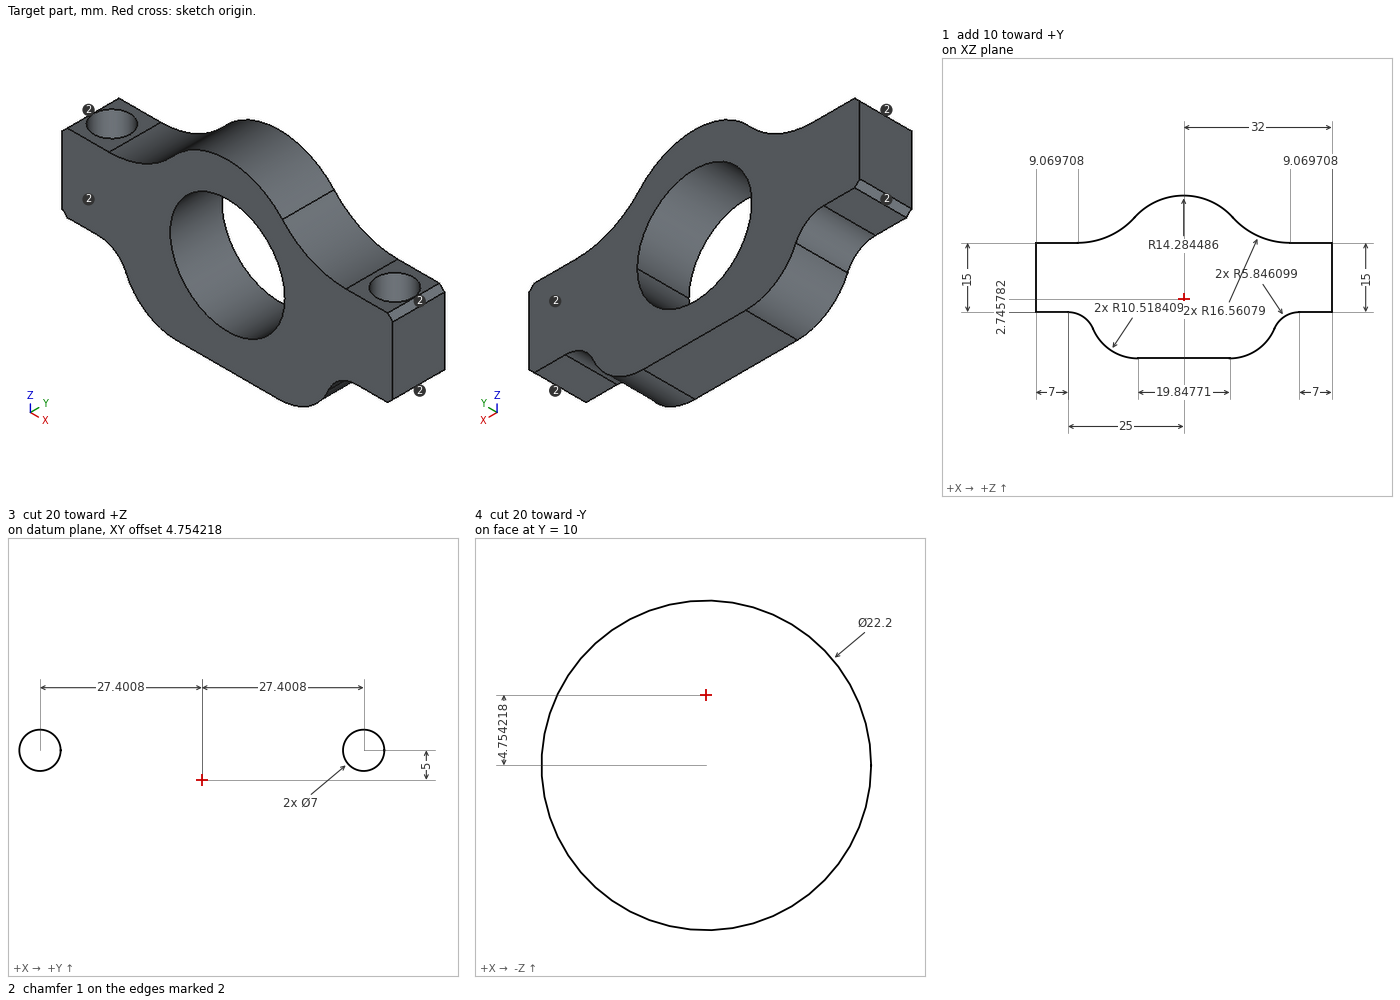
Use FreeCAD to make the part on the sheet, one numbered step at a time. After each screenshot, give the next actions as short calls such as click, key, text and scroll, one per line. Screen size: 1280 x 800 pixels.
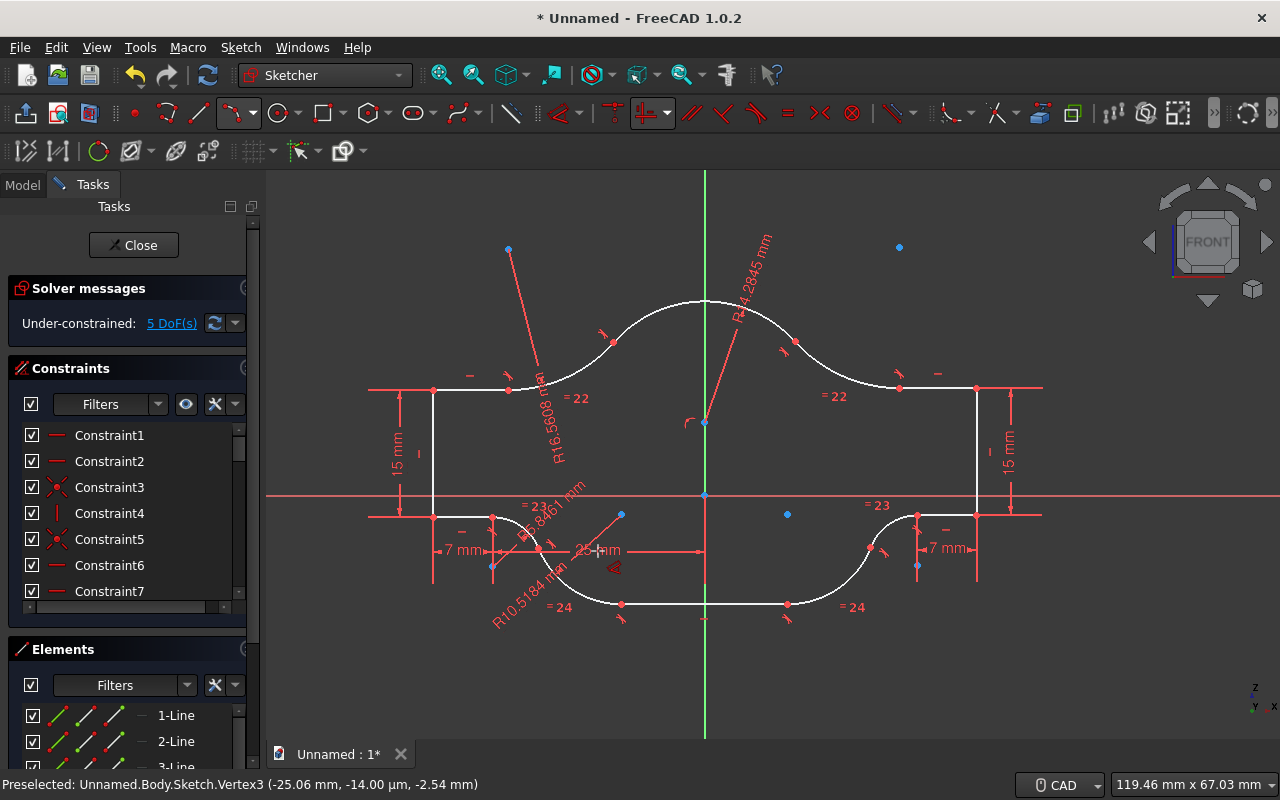
click(977, 388)
click(841, 354)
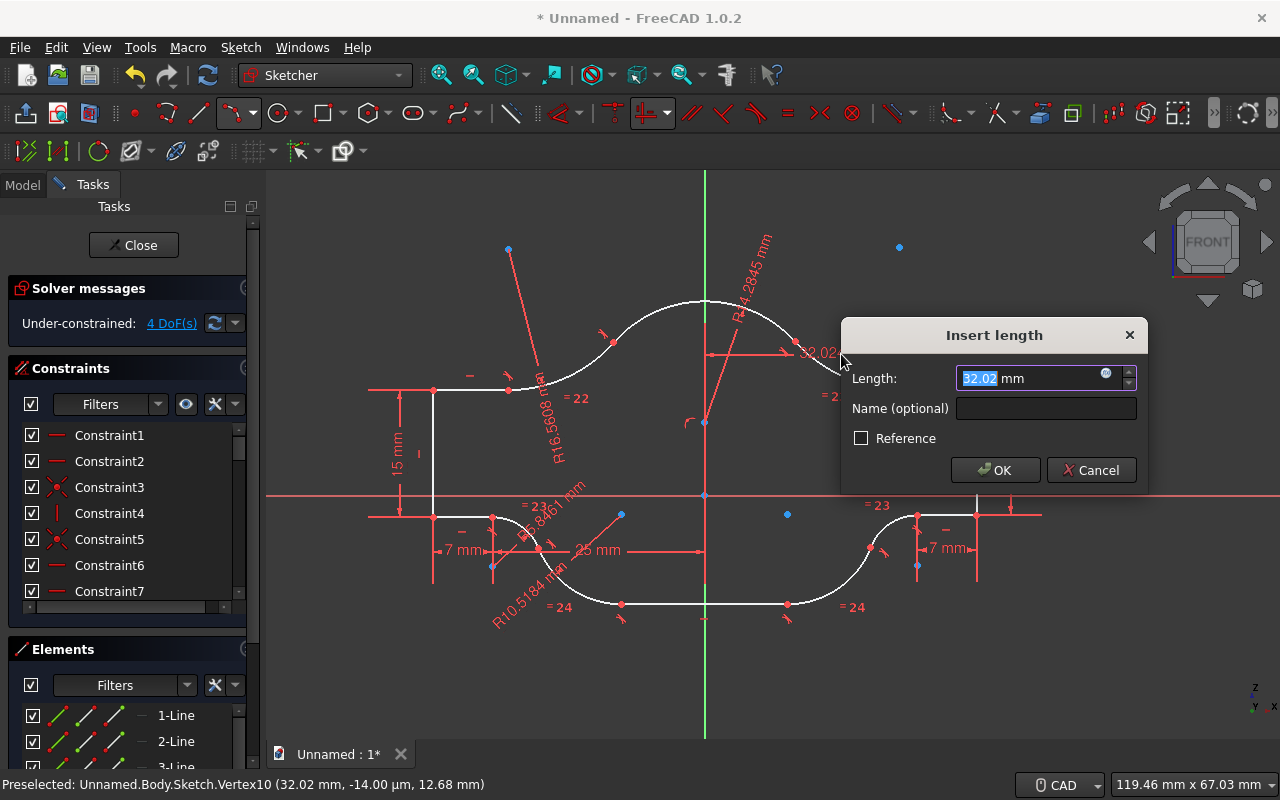
text(32)
key(Return)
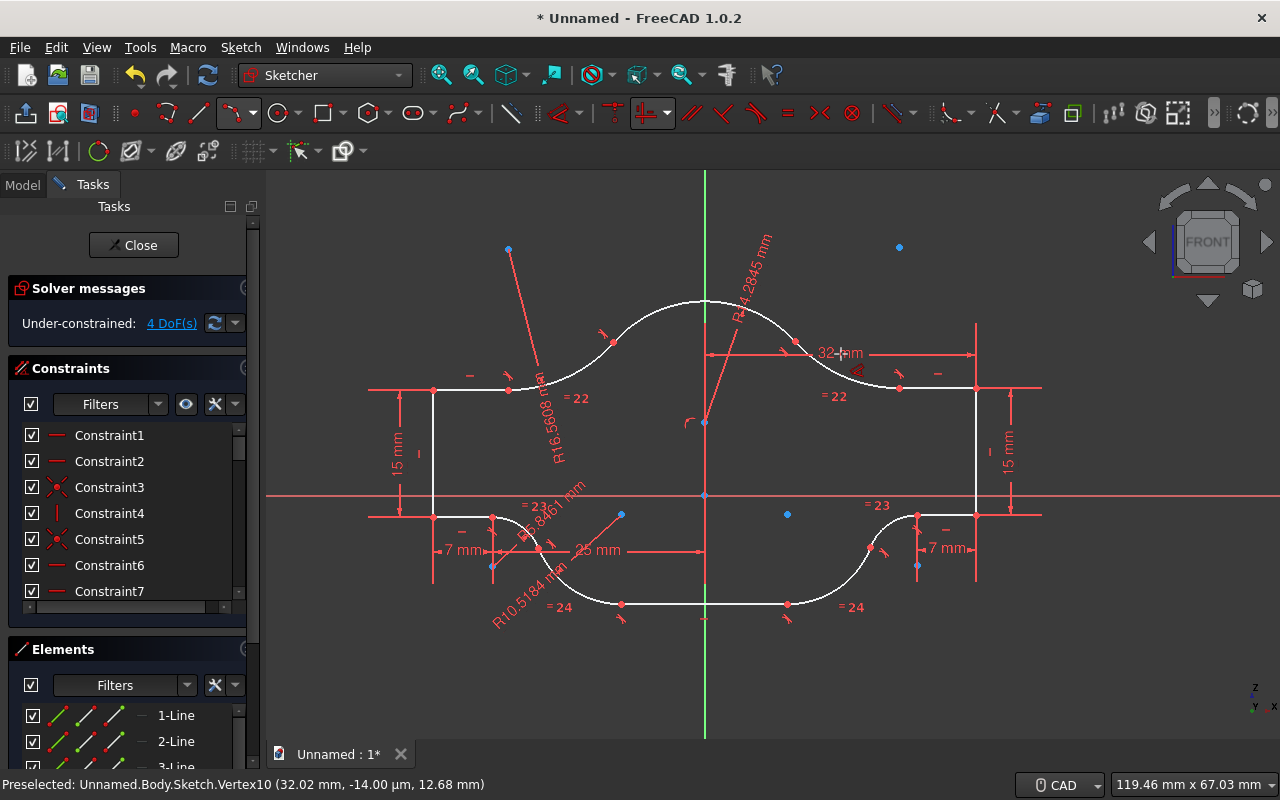
click(738, 604)
click(666, 638)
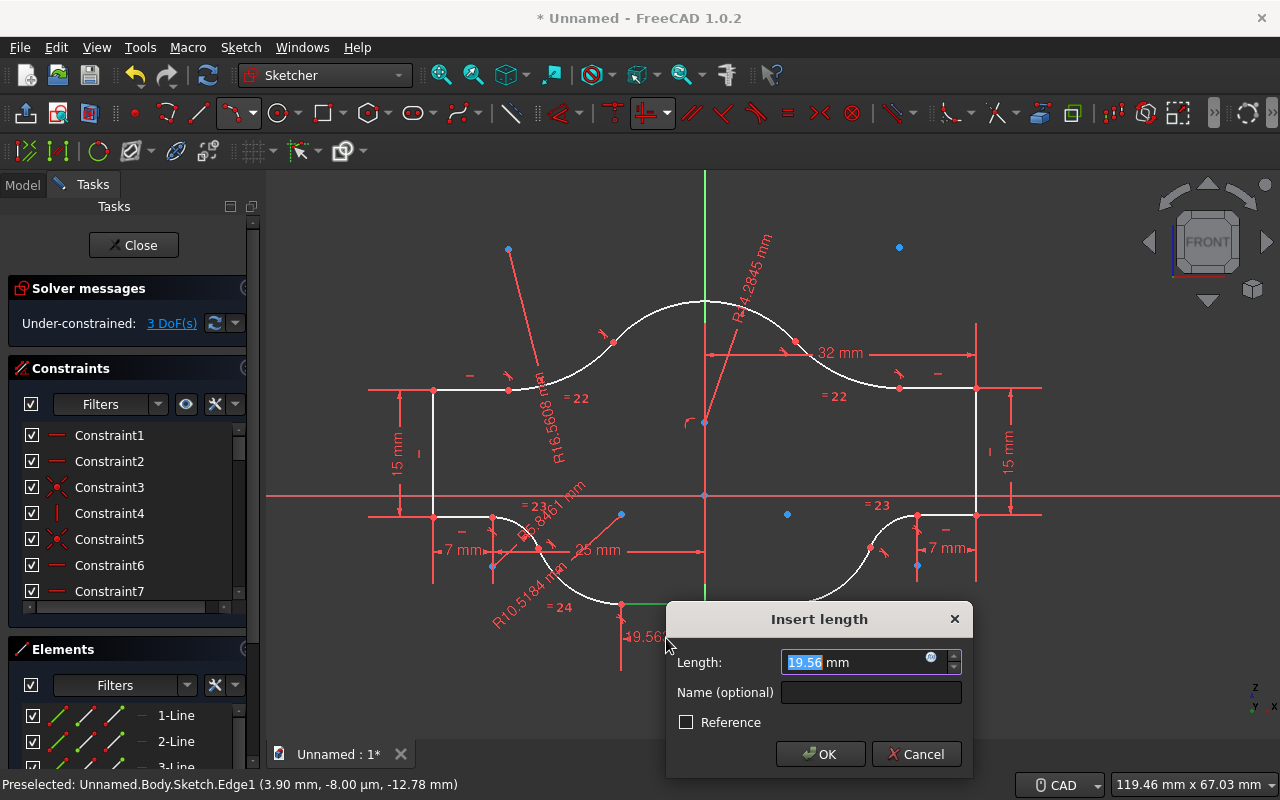
text(19.84771)
key(Return)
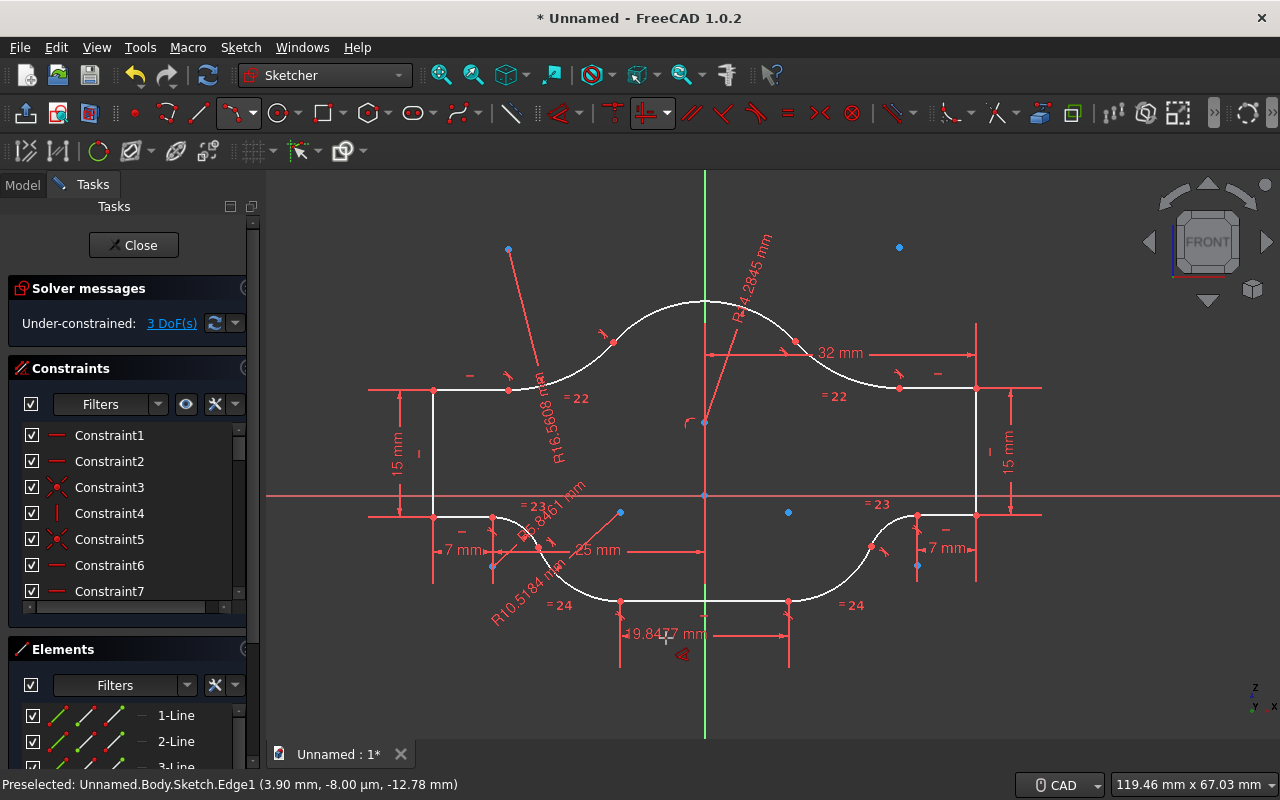
click(456, 390)
click(471, 356)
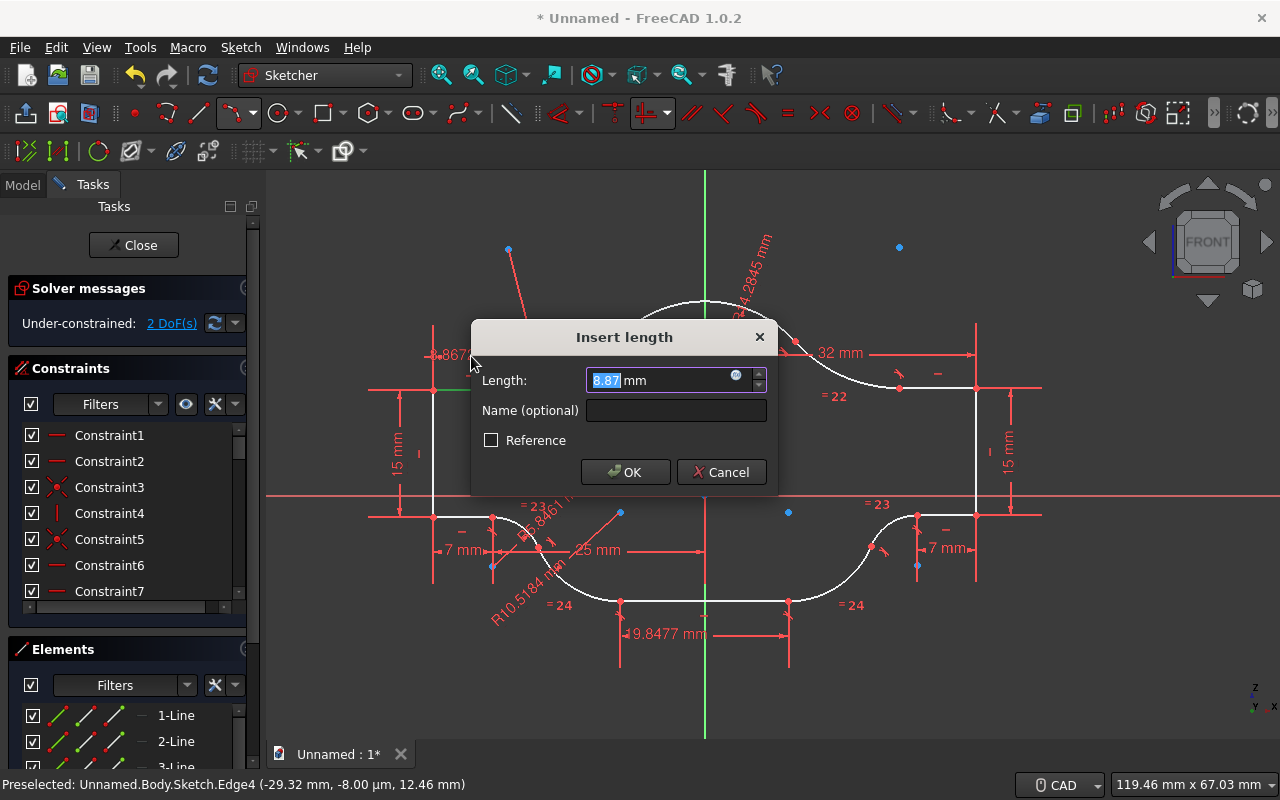
text(9.069708)
key(Return)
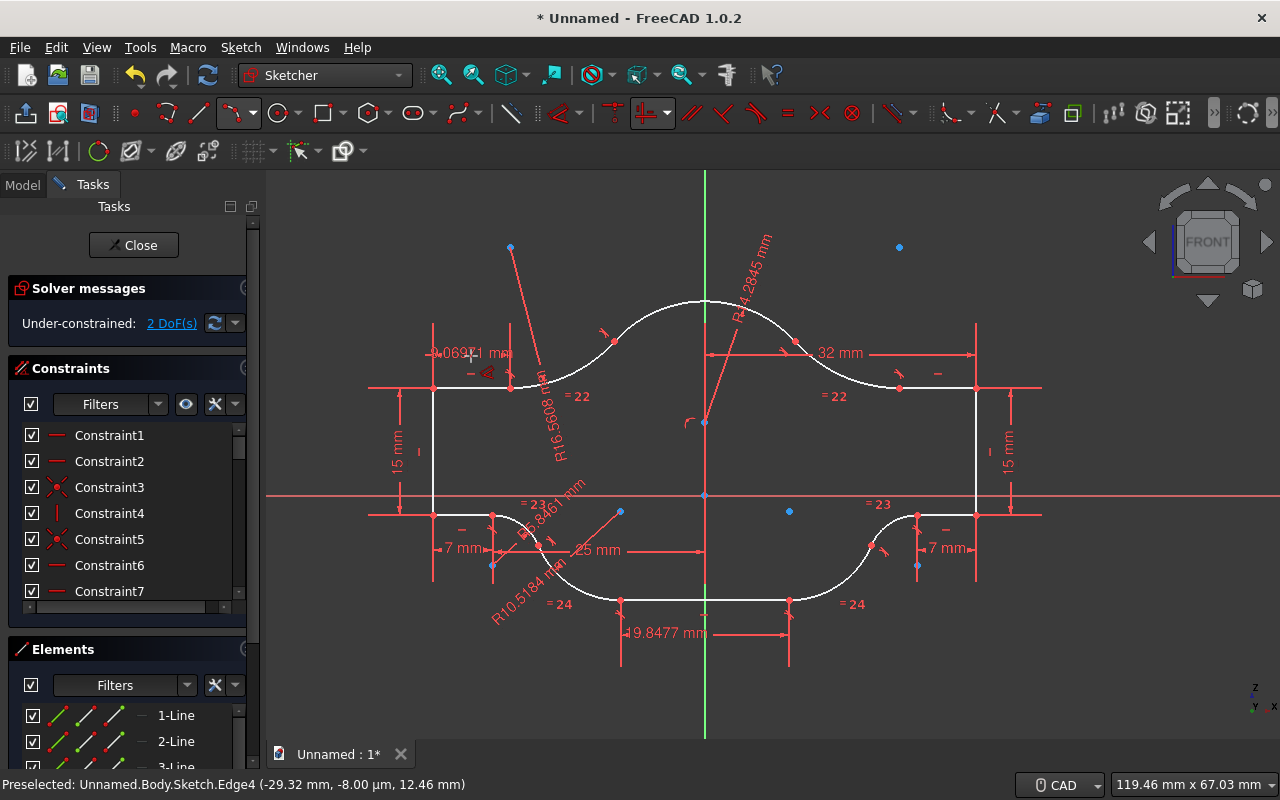
click(923, 388)
click(938, 354)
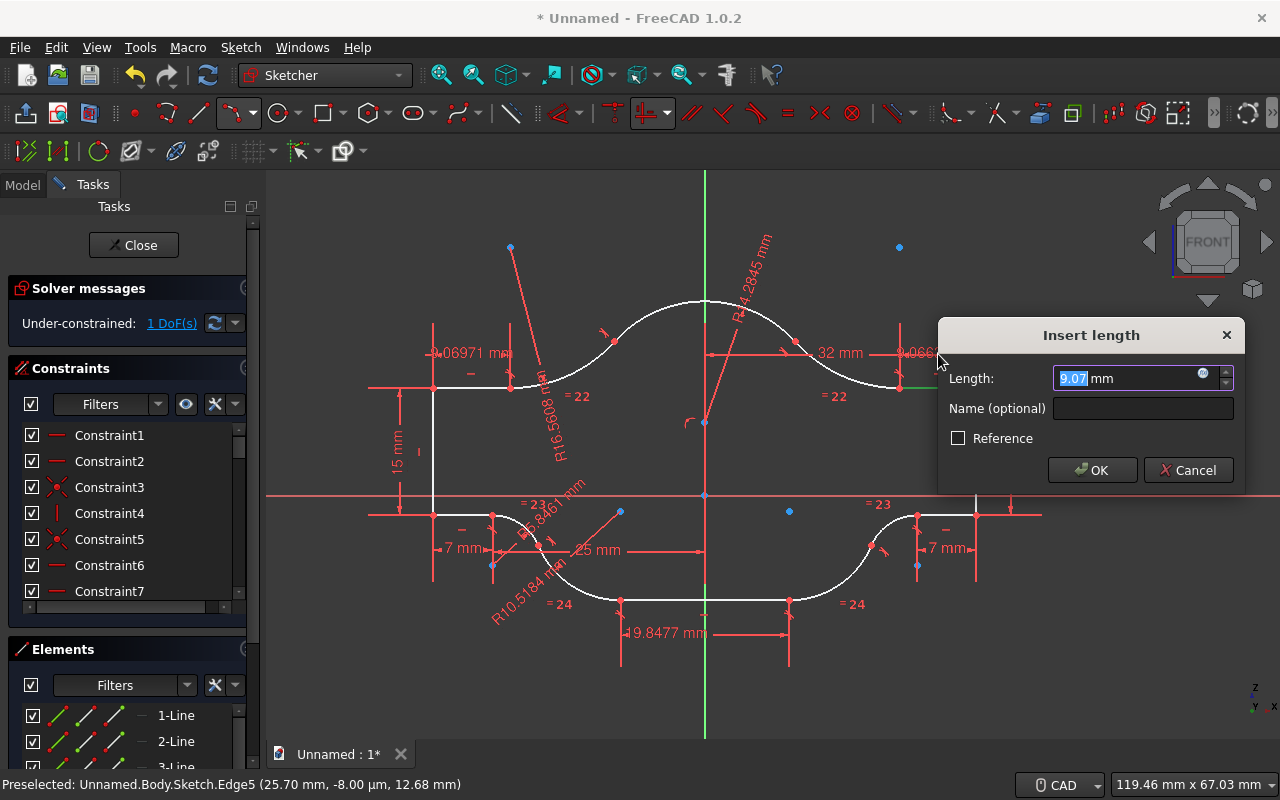
text(9.069708)
key(Return)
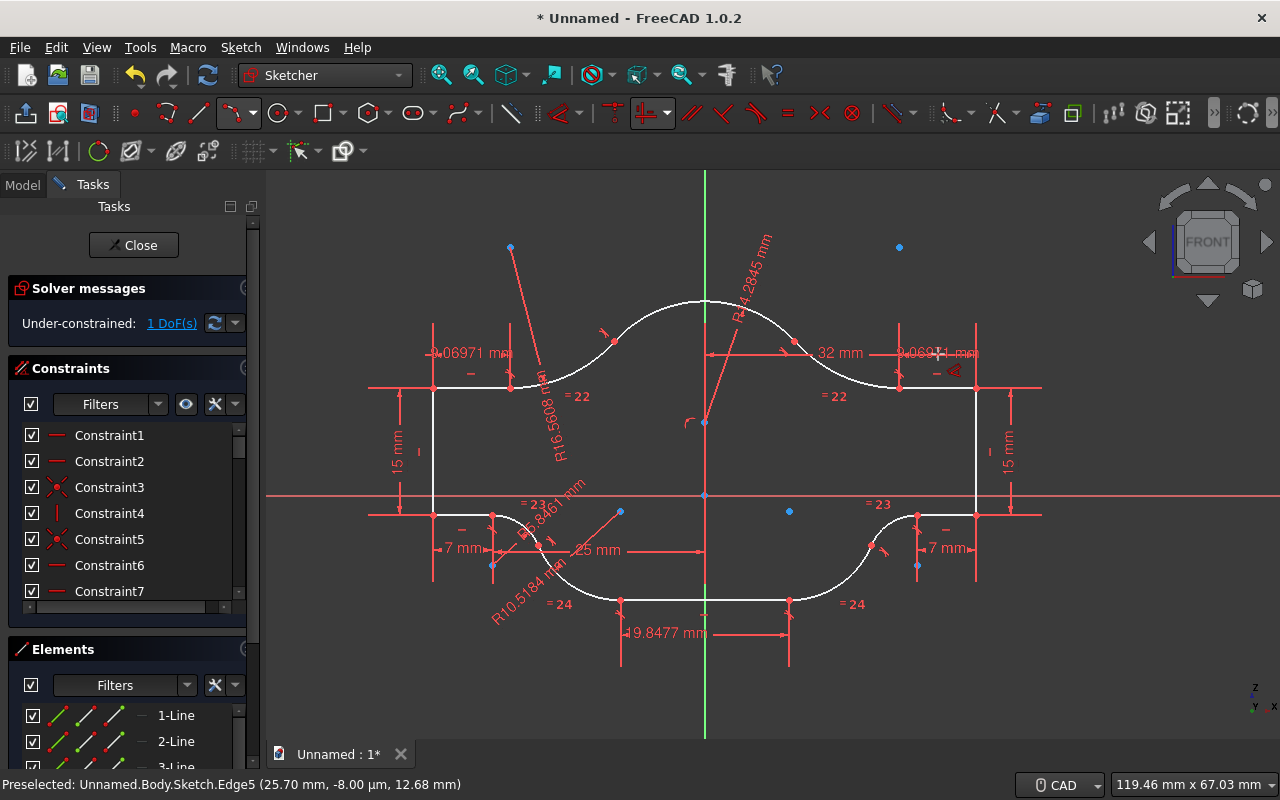
scroll(493, 515, up, 3)